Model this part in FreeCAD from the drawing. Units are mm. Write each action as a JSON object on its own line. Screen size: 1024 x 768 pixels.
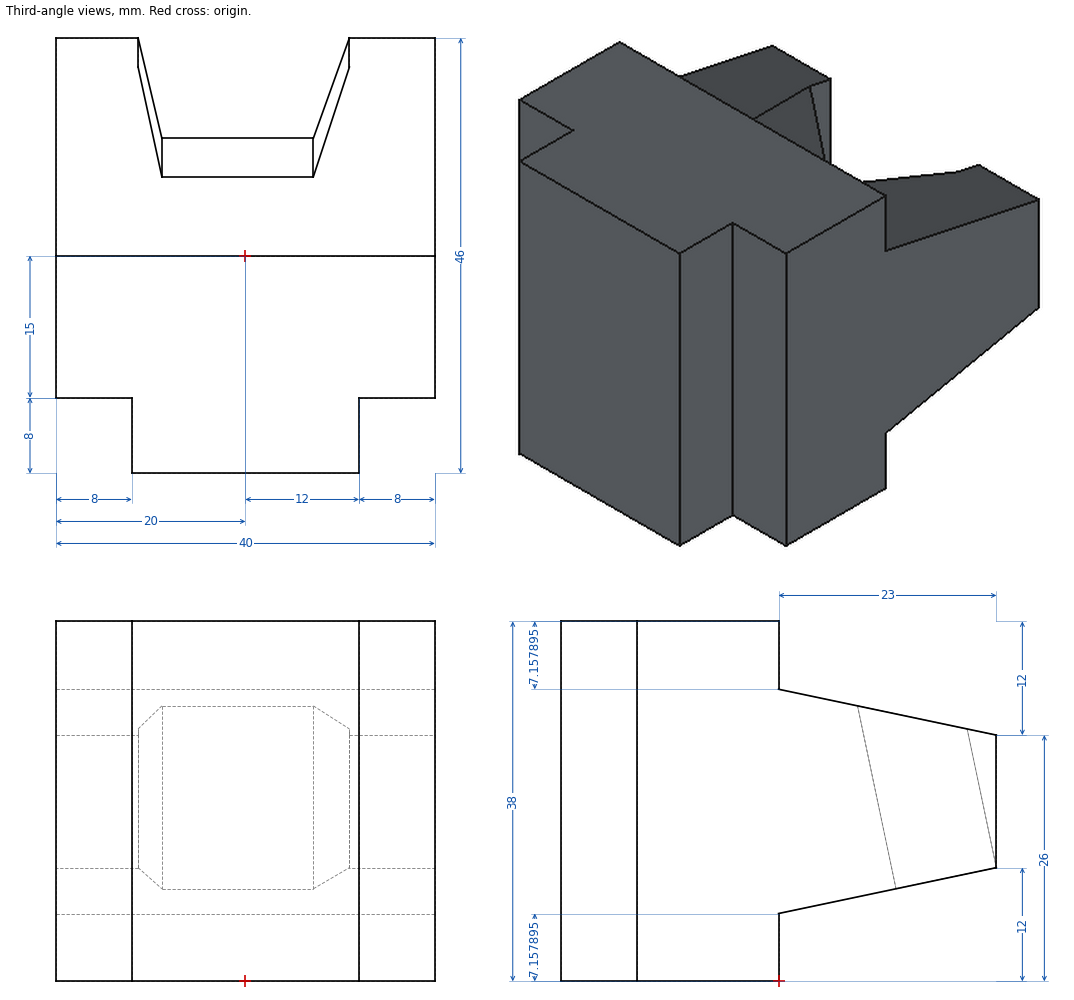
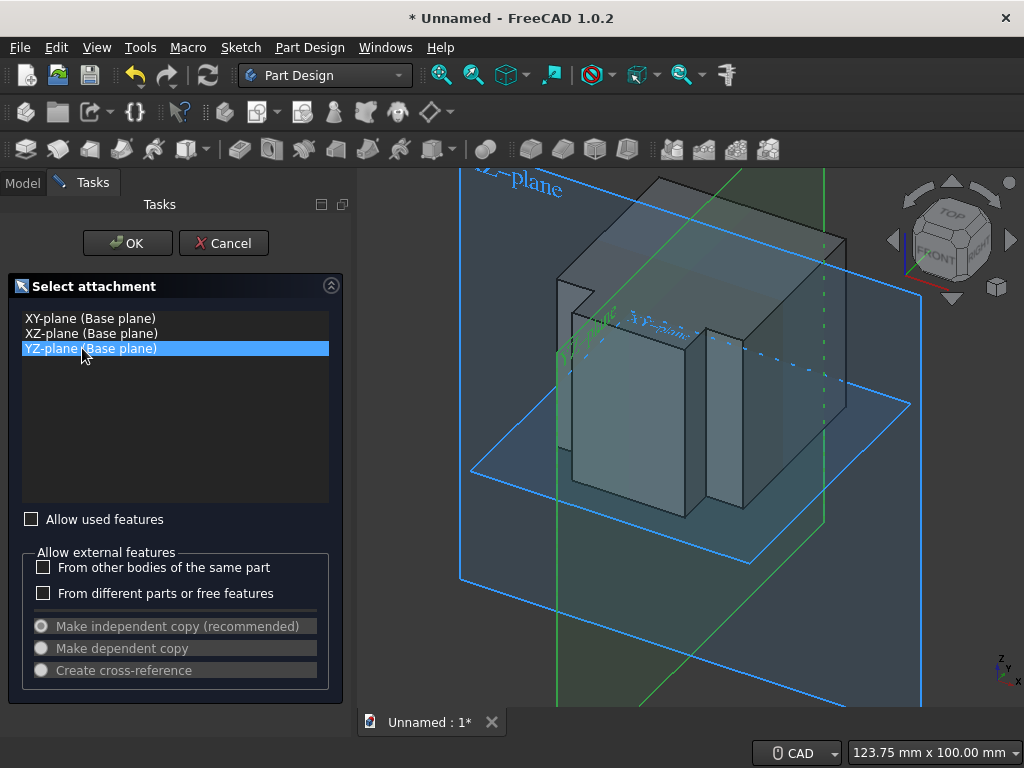
{"action": "left_click", "coordinate": [128, 243]}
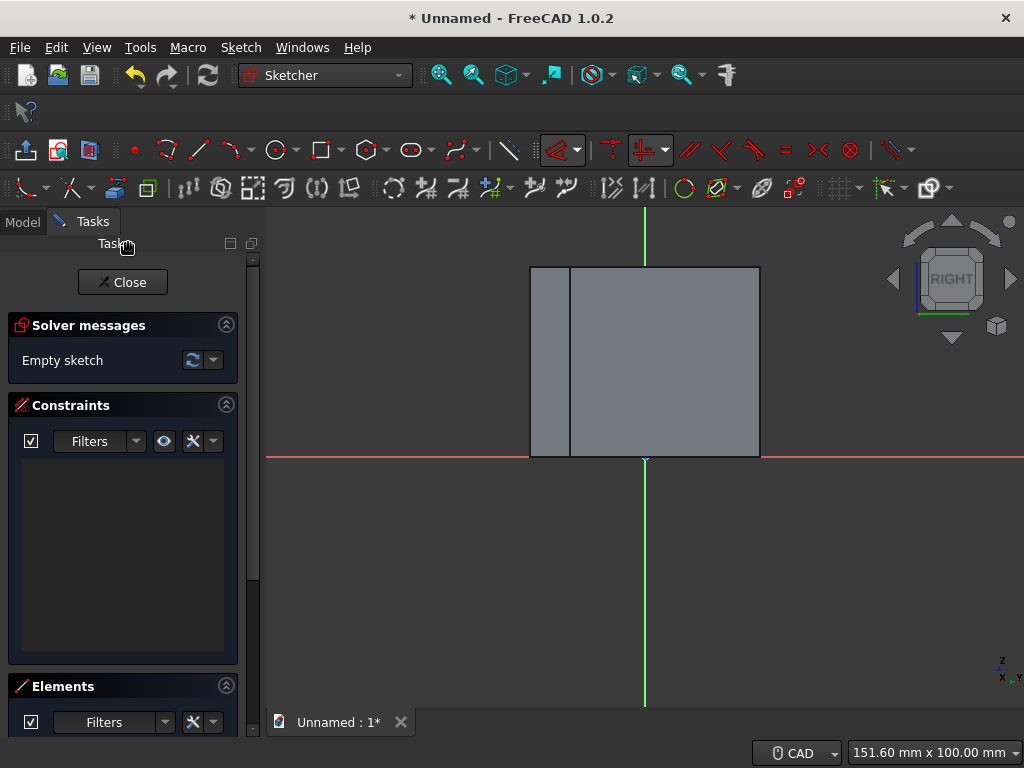
{"action": "left_click", "coordinate": [90, 150]}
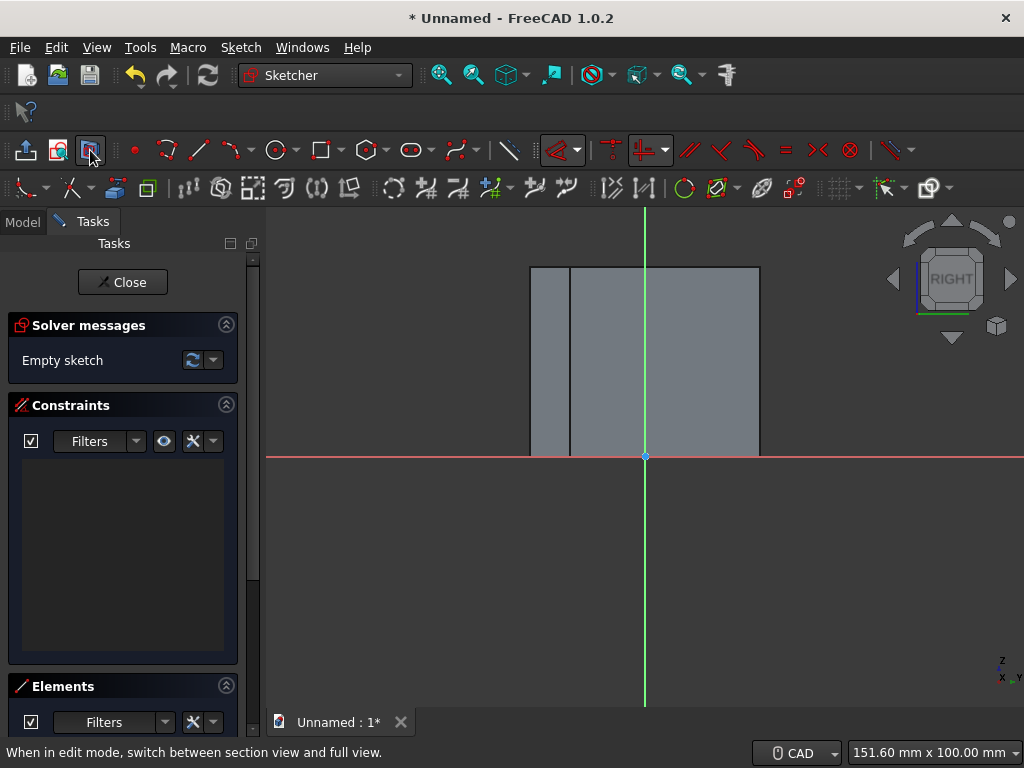
{"action": "scroll", "coordinate": [856, 246], "scroll_direction": "up", "scroll_amount": 3}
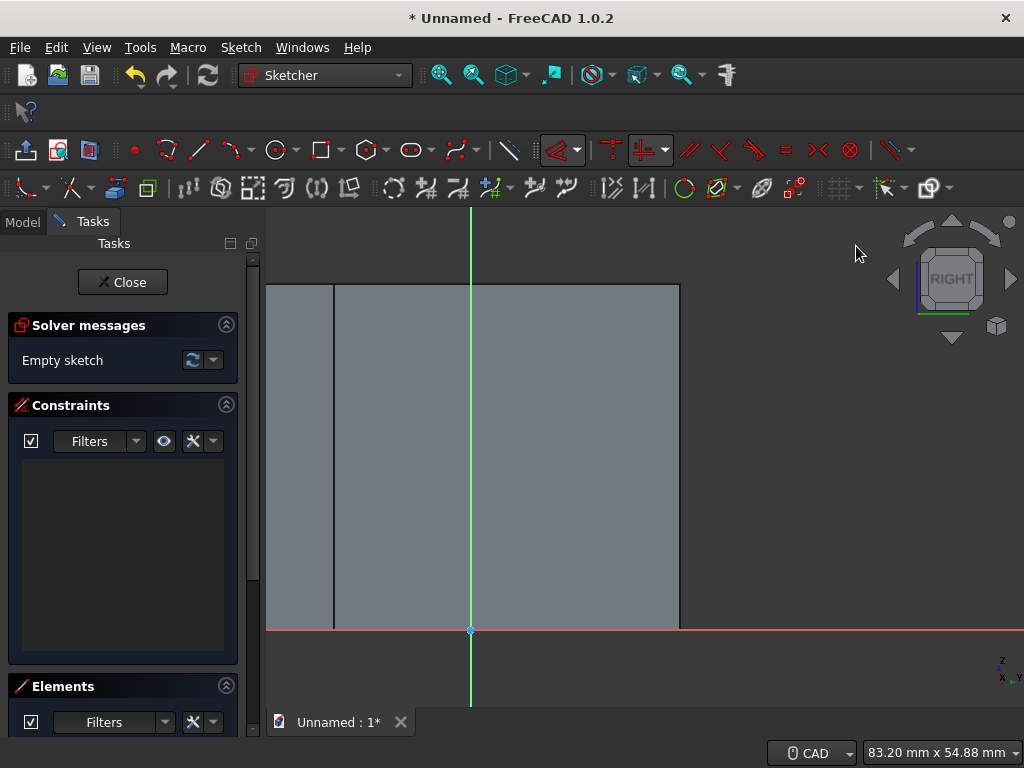
{"action": "left_click", "coordinate": [168, 150]}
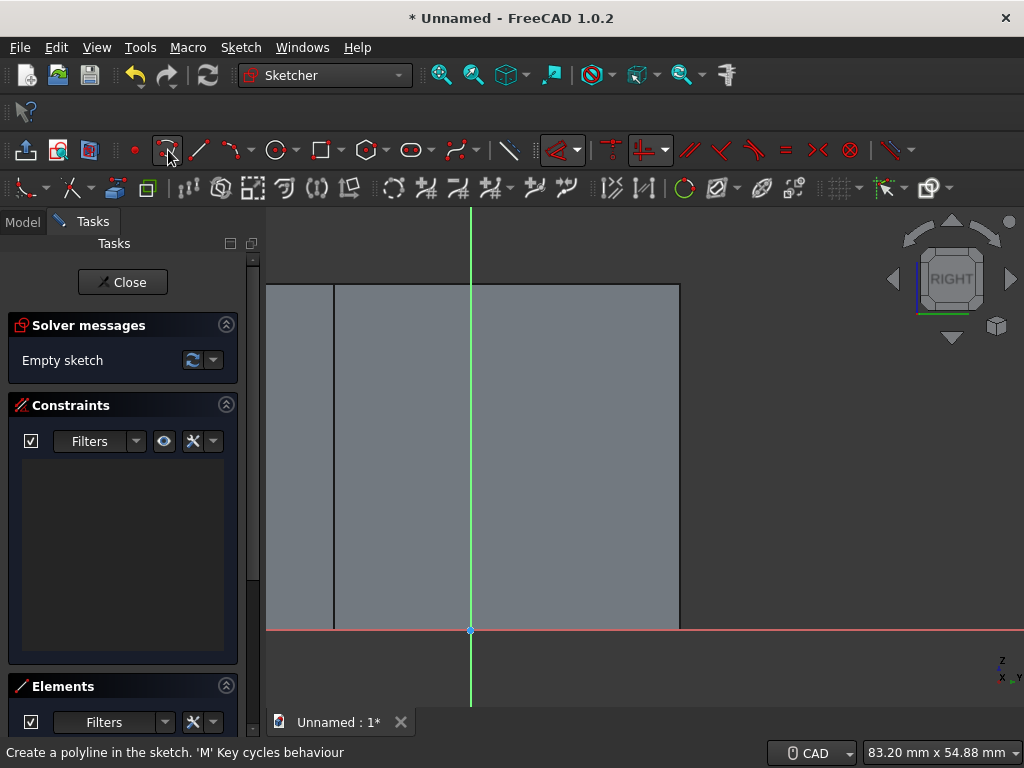
{"action": "left_click", "coordinate": [471, 349]}
{"action": "left_click", "coordinate": [680, 394]}
{"action": "left_click", "coordinate": [680, 284]}
{"action": "left_click", "coordinate": [480, 284]}
{"action": "left_click", "coordinate": [471, 350]}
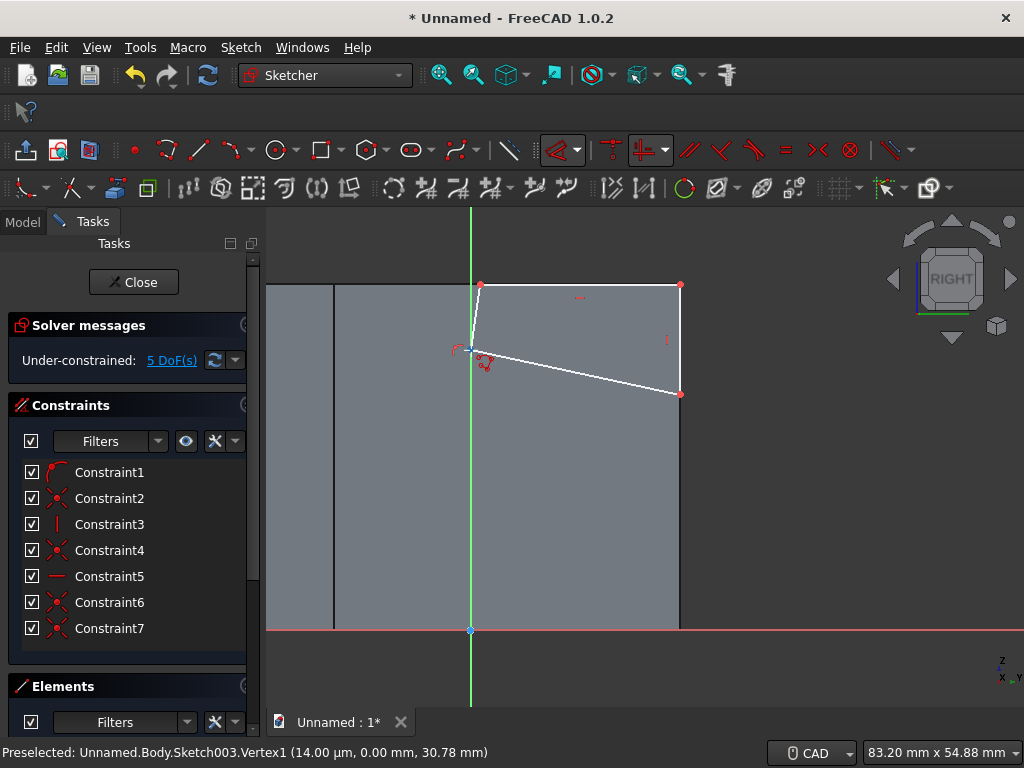
{"action": "left_click", "coordinate": [471, 630]}
{"action": "left_click", "coordinate": [680, 621]}
{"action": "left_click", "coordinate": [680, 521]}
{"action": "left_click", "coordinate": [480, 565]}
{"action": "left_click", "coordinate": [471, 630]}
{"action": "key", "text": "Escape"}
{"action": "key", "text": "Escape"}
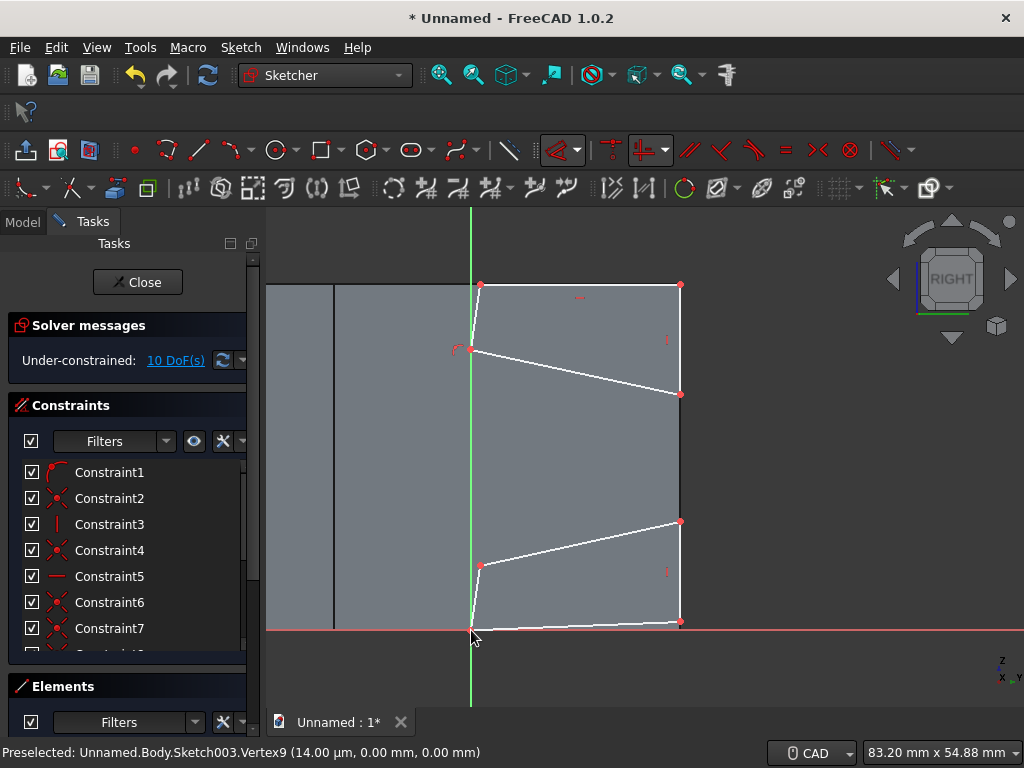
{"action": "left_click", "coordinate": [474, 331]}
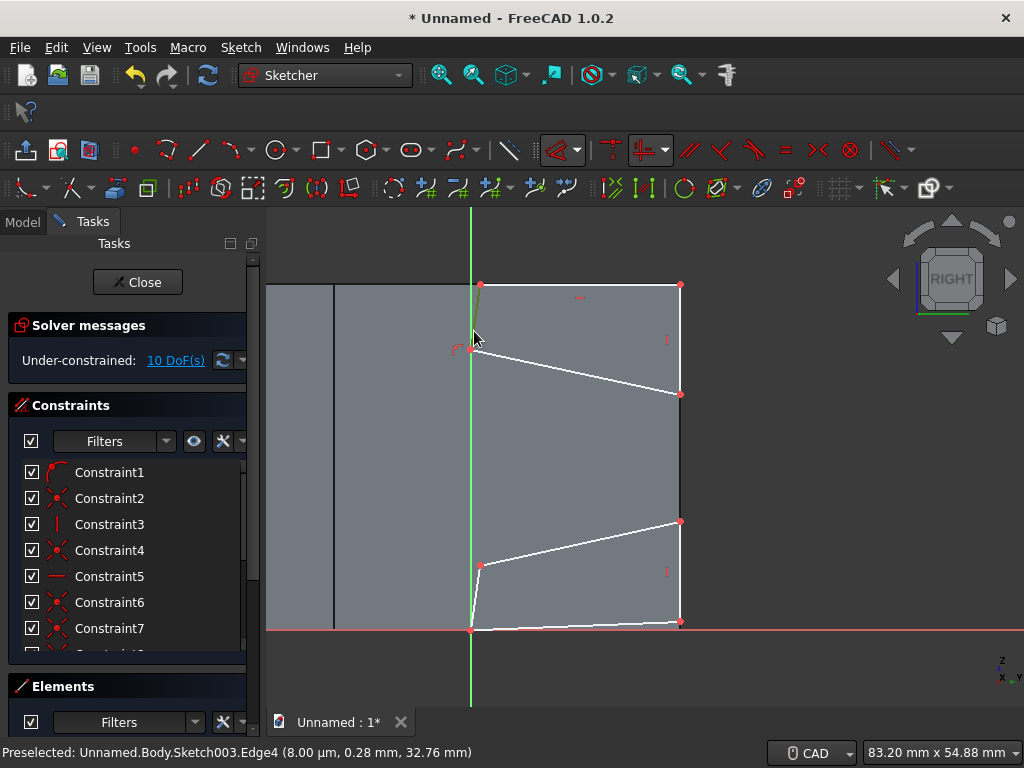
{"action": "key", "text": "v"}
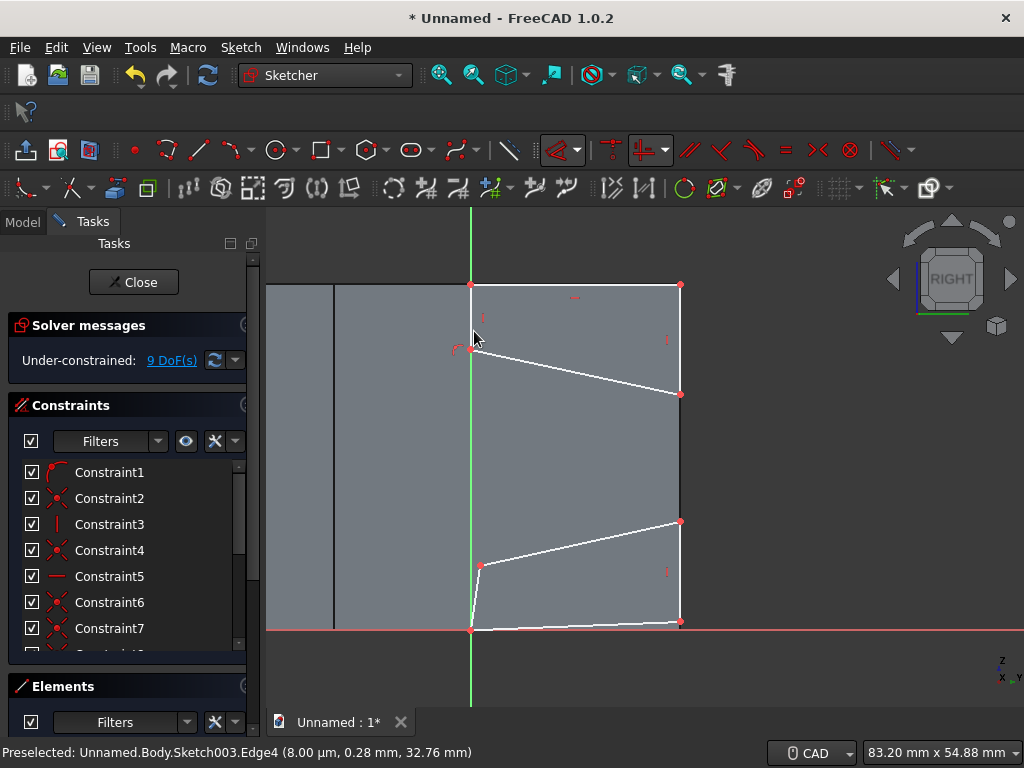
{"action": "left_click", "coordinate": [534, 628]}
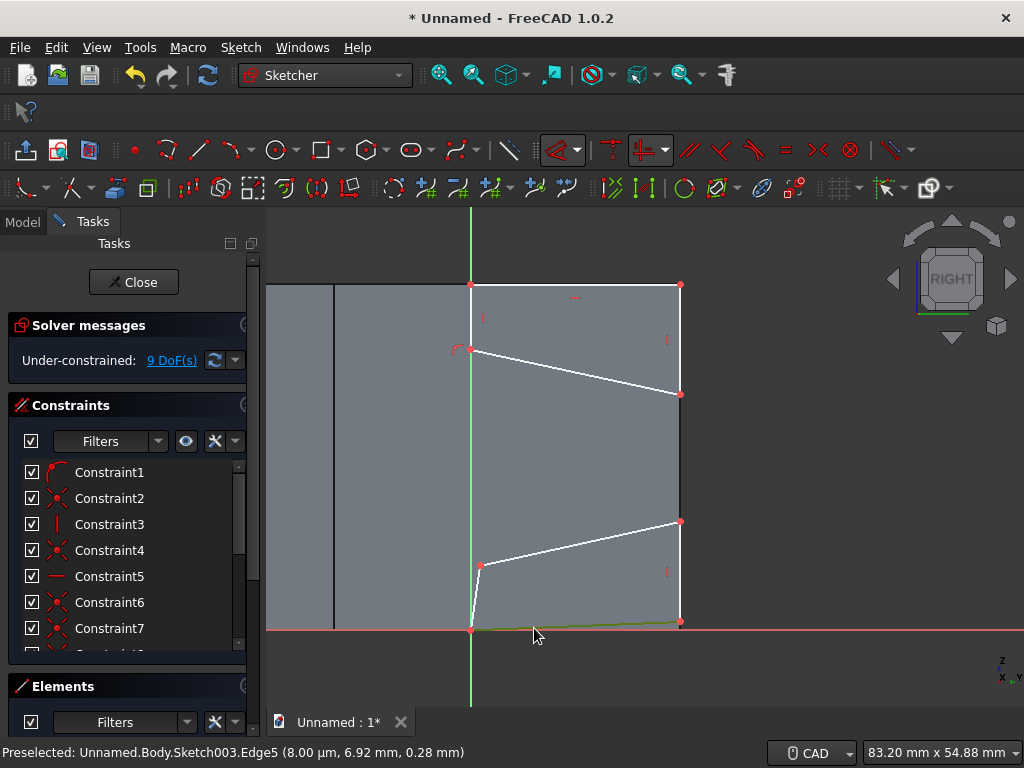
{"action": "key", "text": "h"}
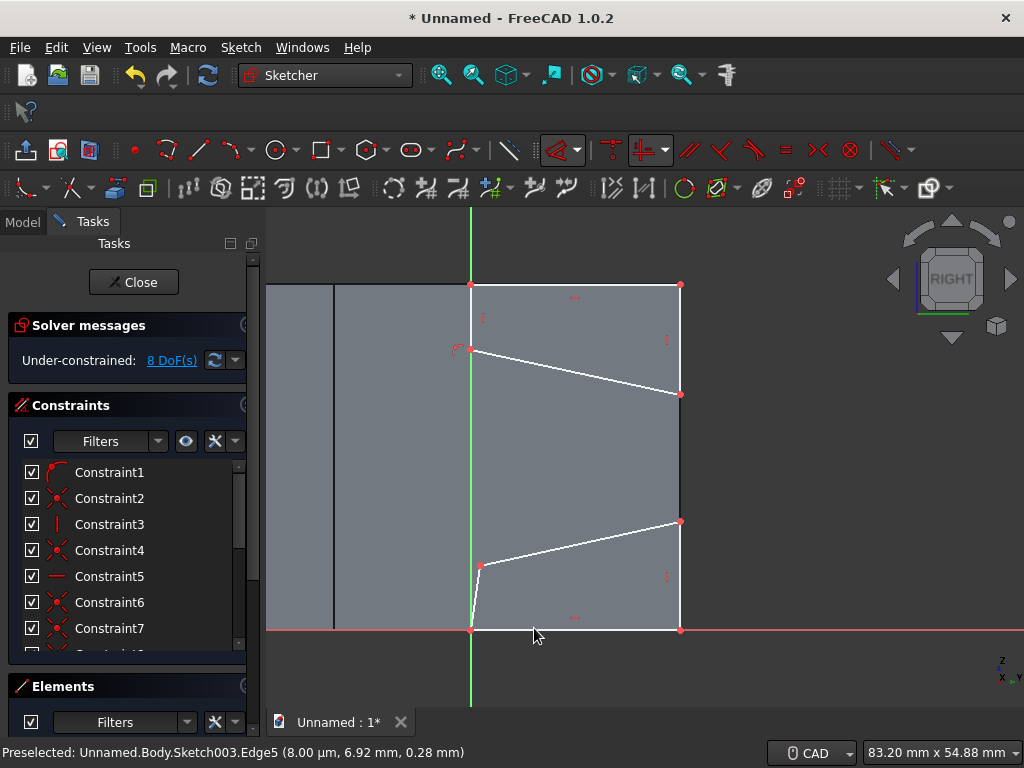
{"action": "left_click", "coordinate": [474, 611]}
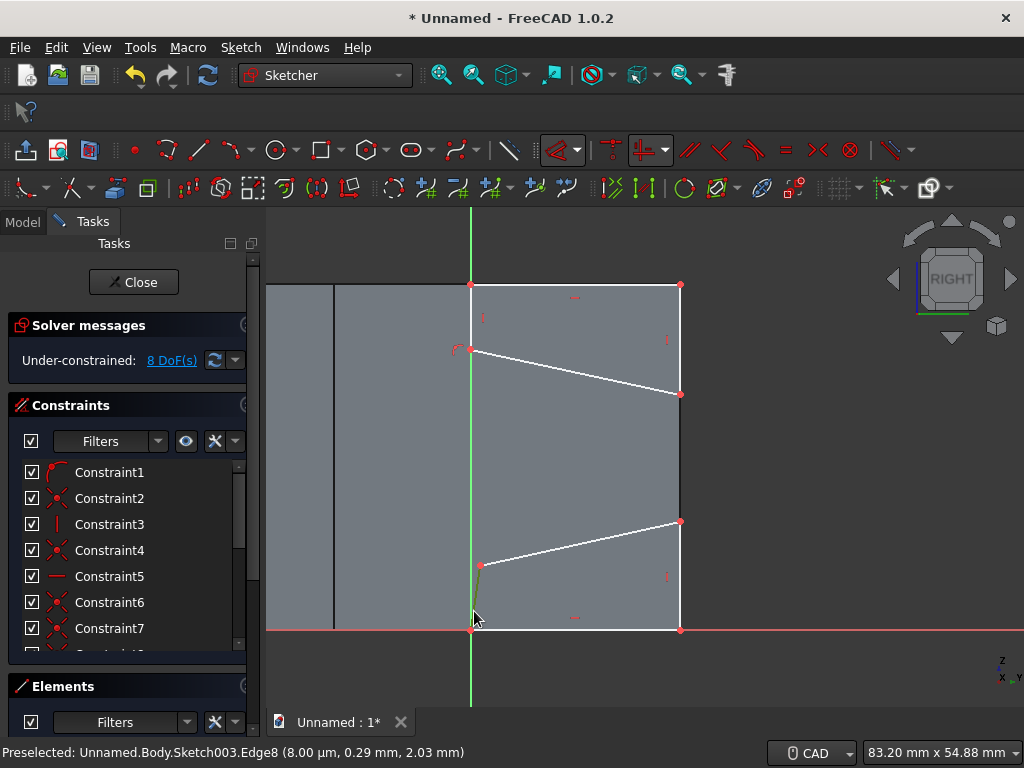
{"action": "left_click", "coordinate": [668, 150]}